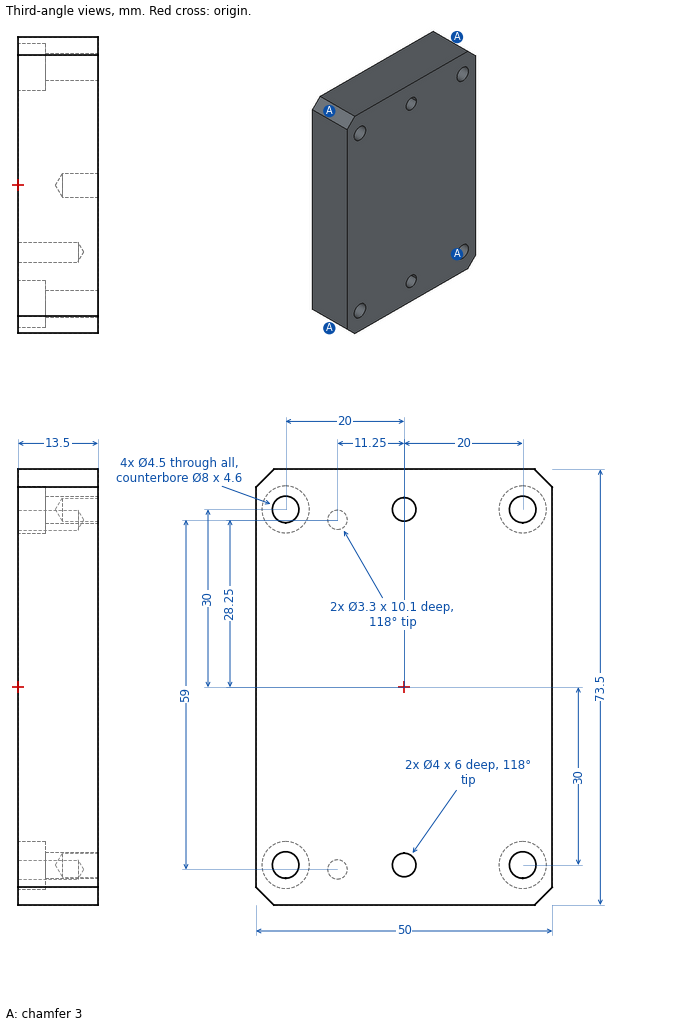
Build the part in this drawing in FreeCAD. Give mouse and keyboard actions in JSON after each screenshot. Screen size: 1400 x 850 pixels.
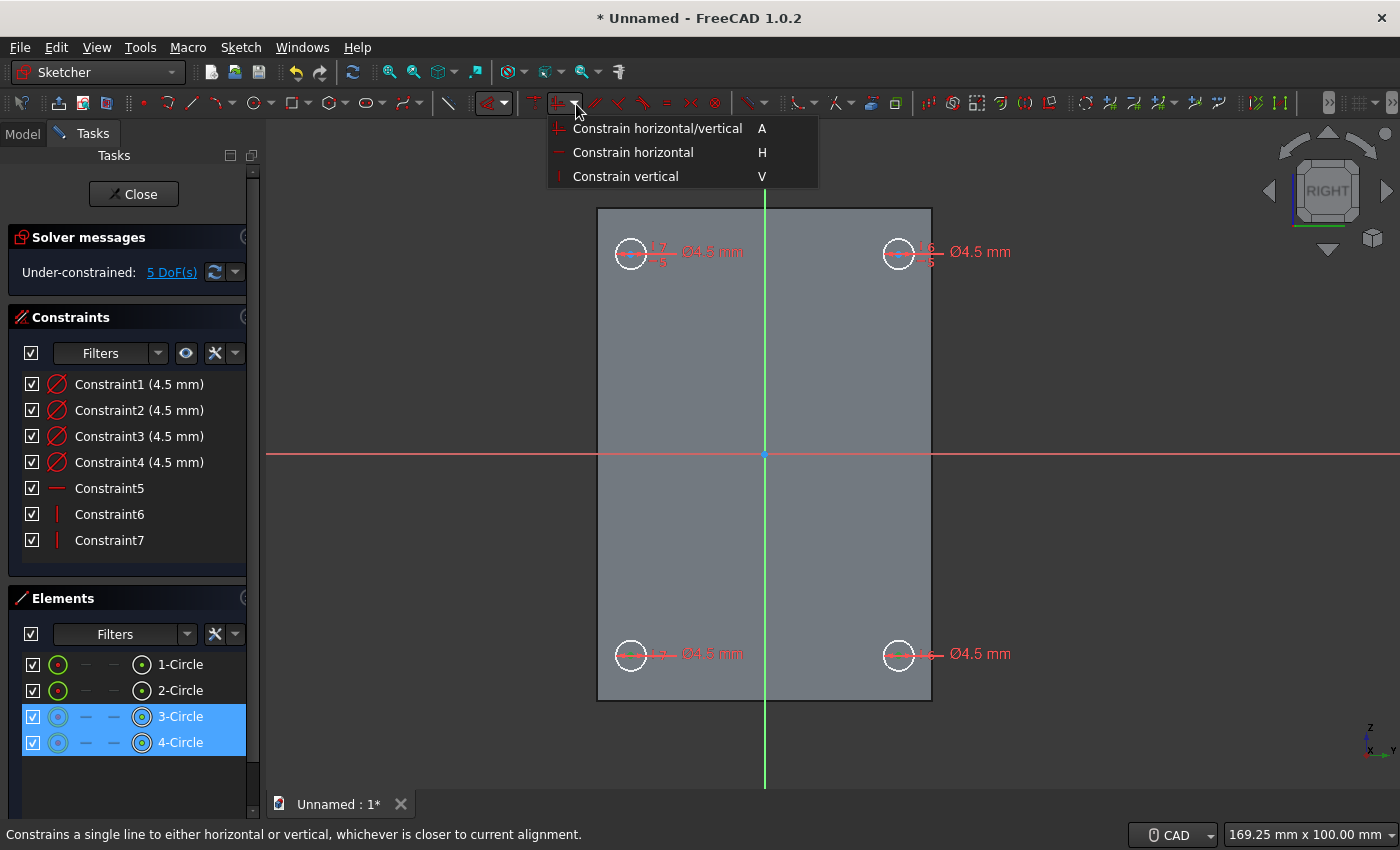
{"action": "left_click", "coordinate": [683, 152]}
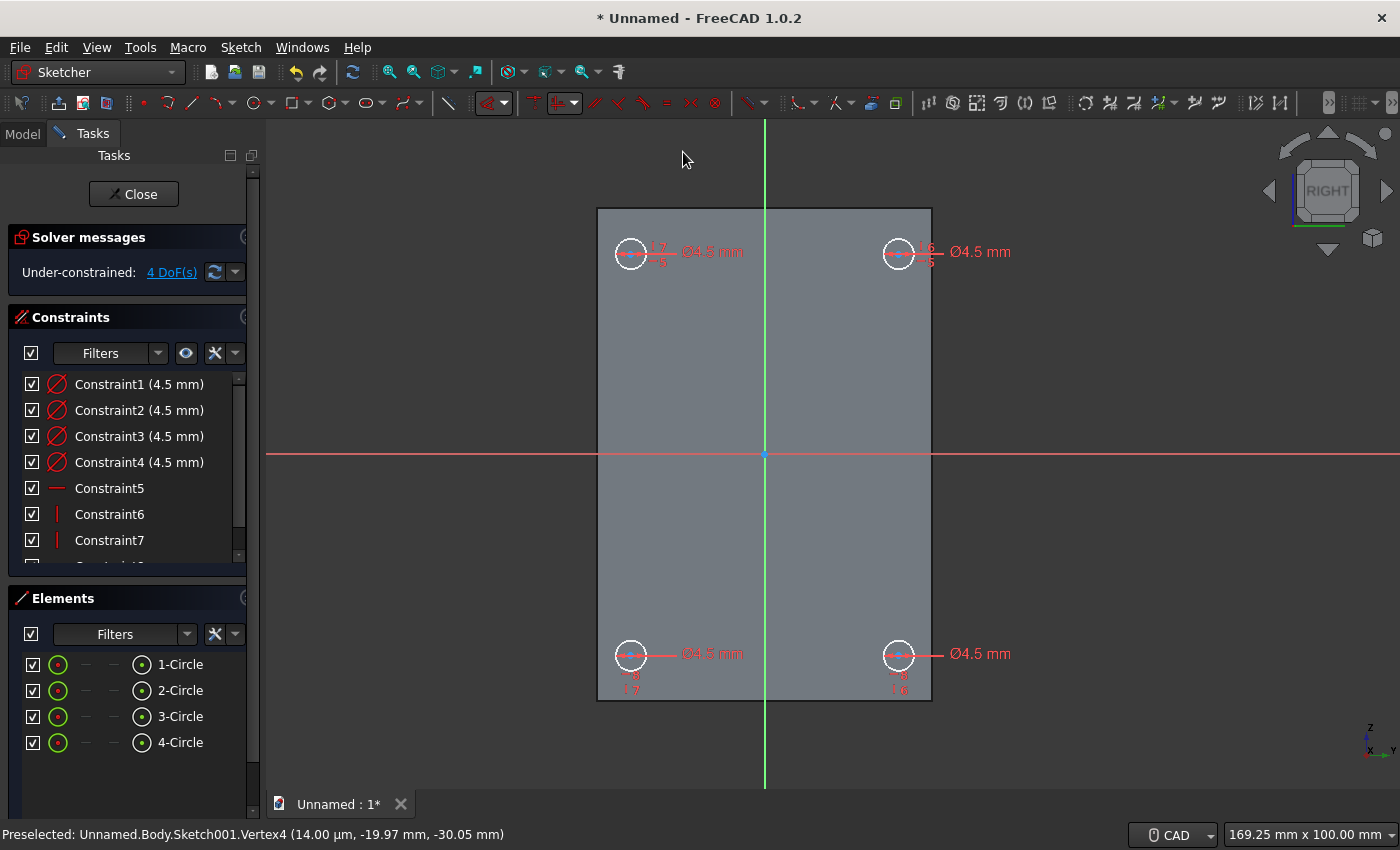
{"action": "left_click", "coordinate": [631, 254]}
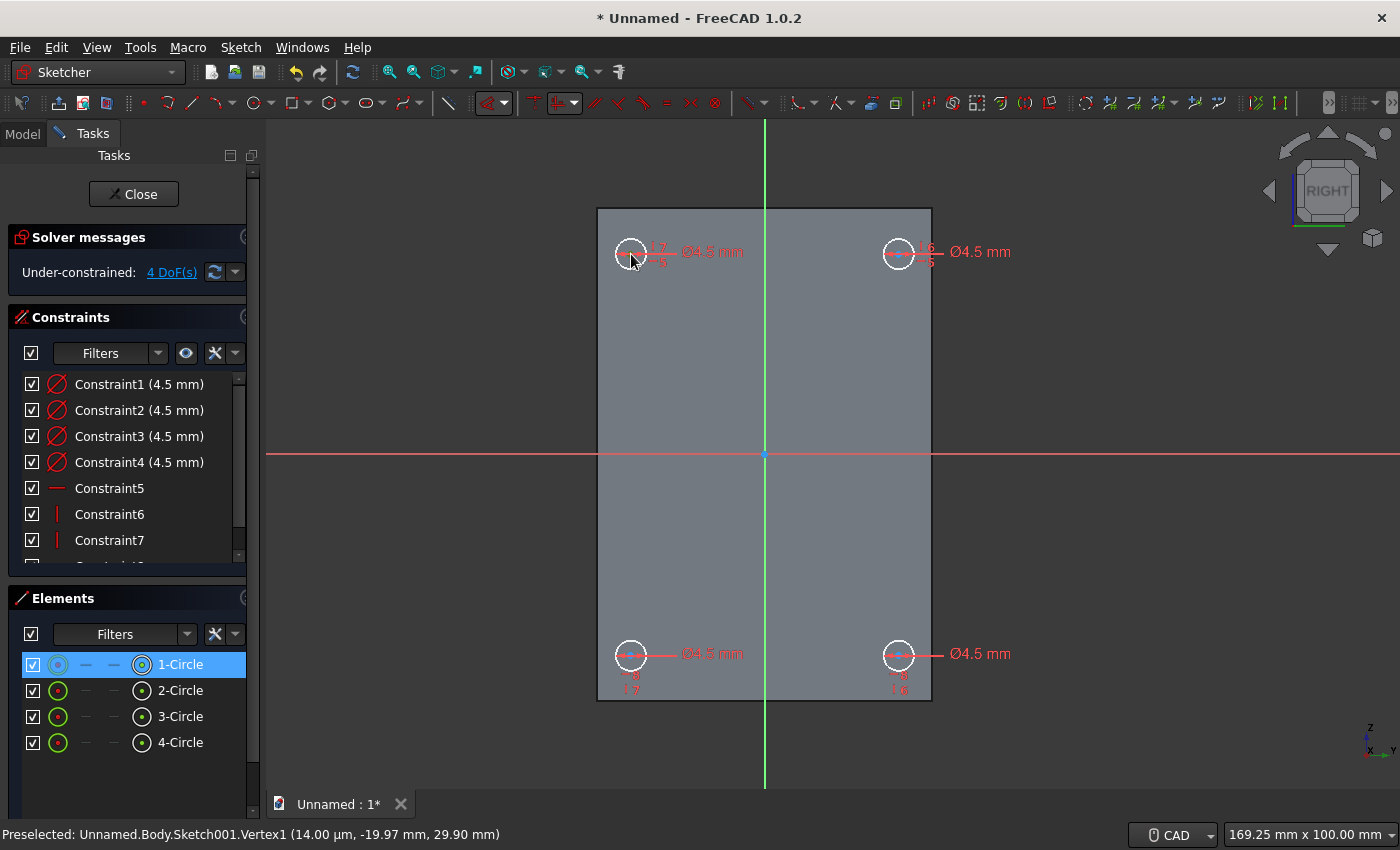
{"action": "left_click", "coordinate": [506, 104]}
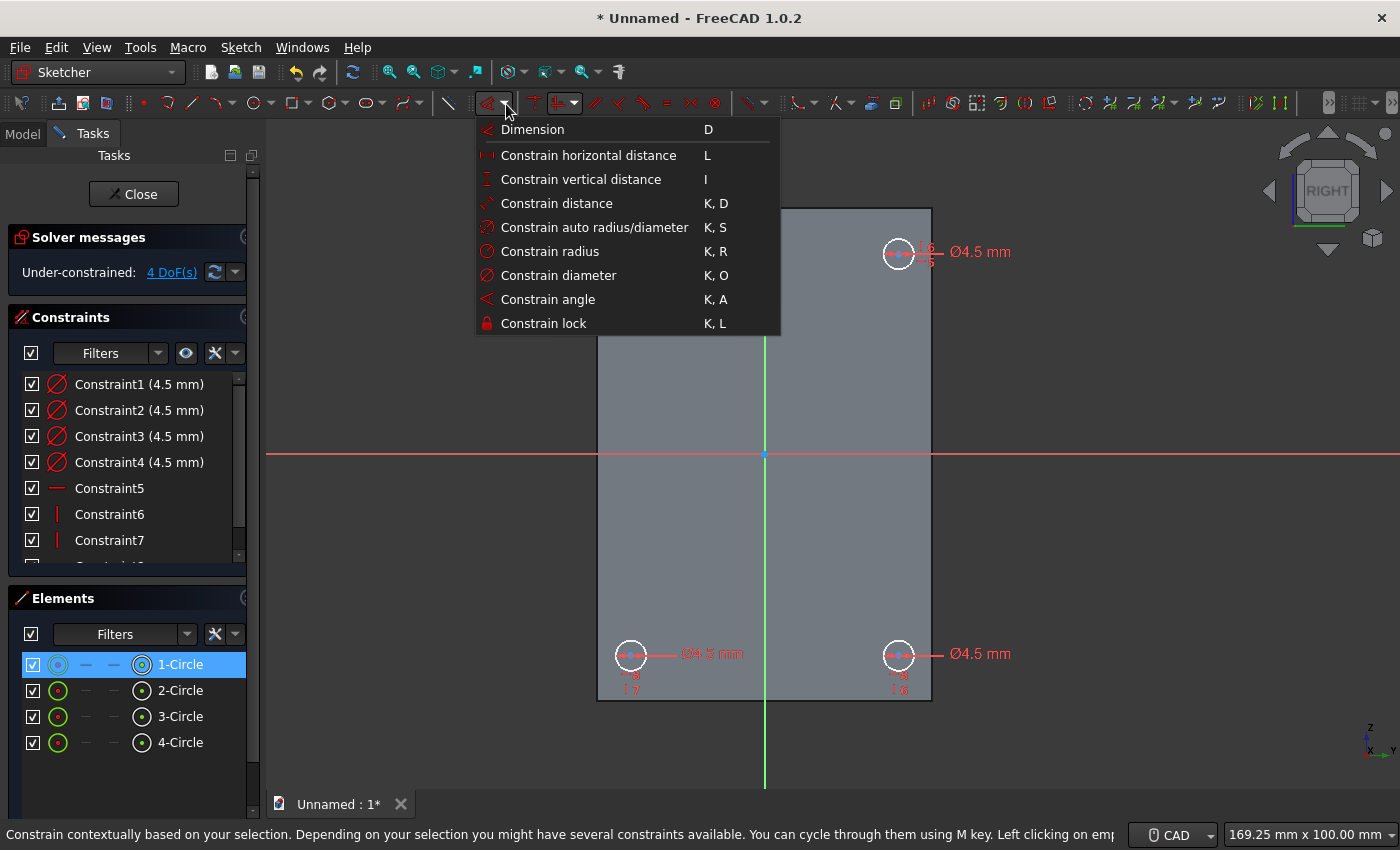
{"action": "left_click", "coordinate": [628, 155]}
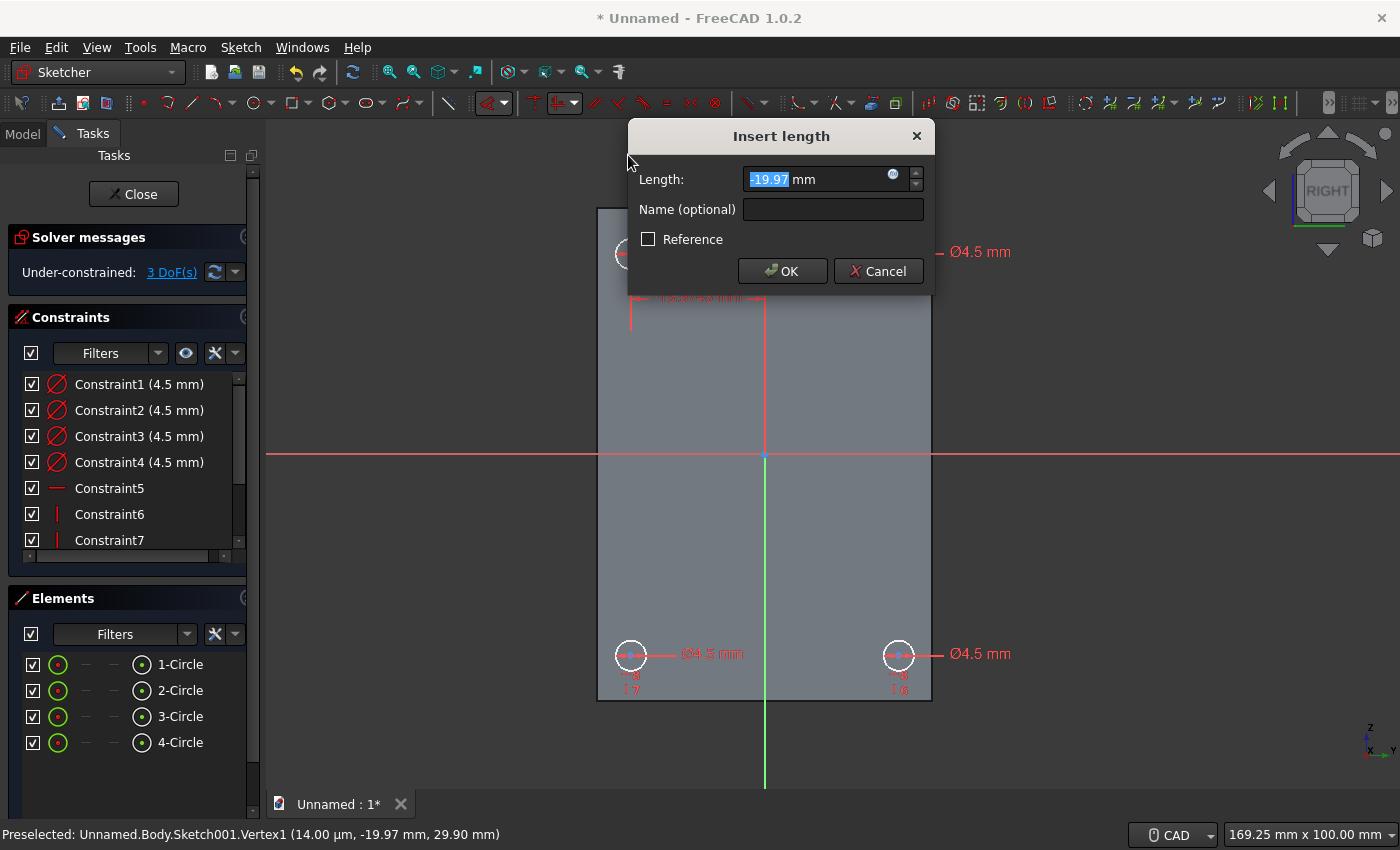
{"action": "type", "text": "-20"}
{"action": "key", "text": "Return"}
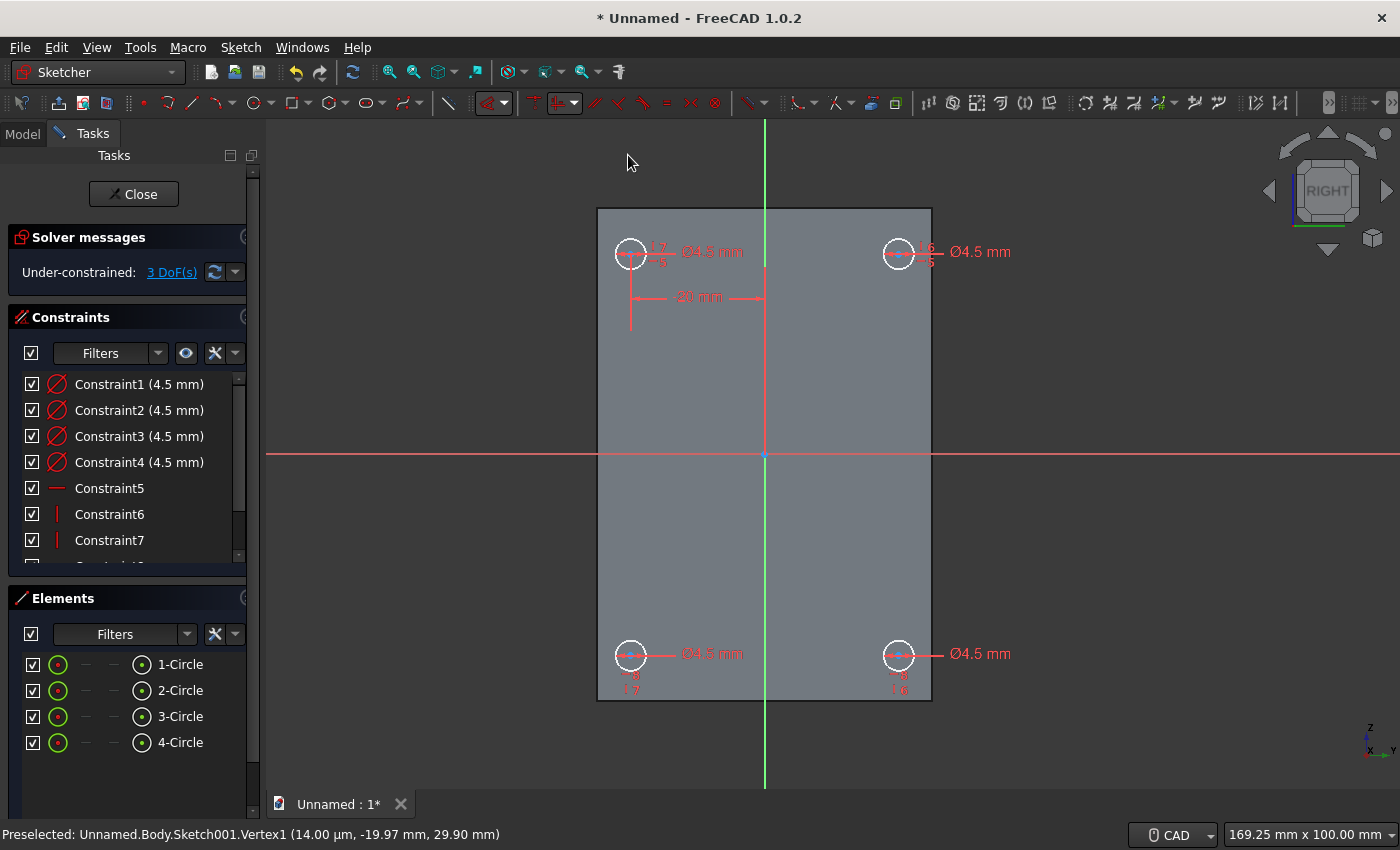
{"action": "left_click", "coordinate": [631, 254]}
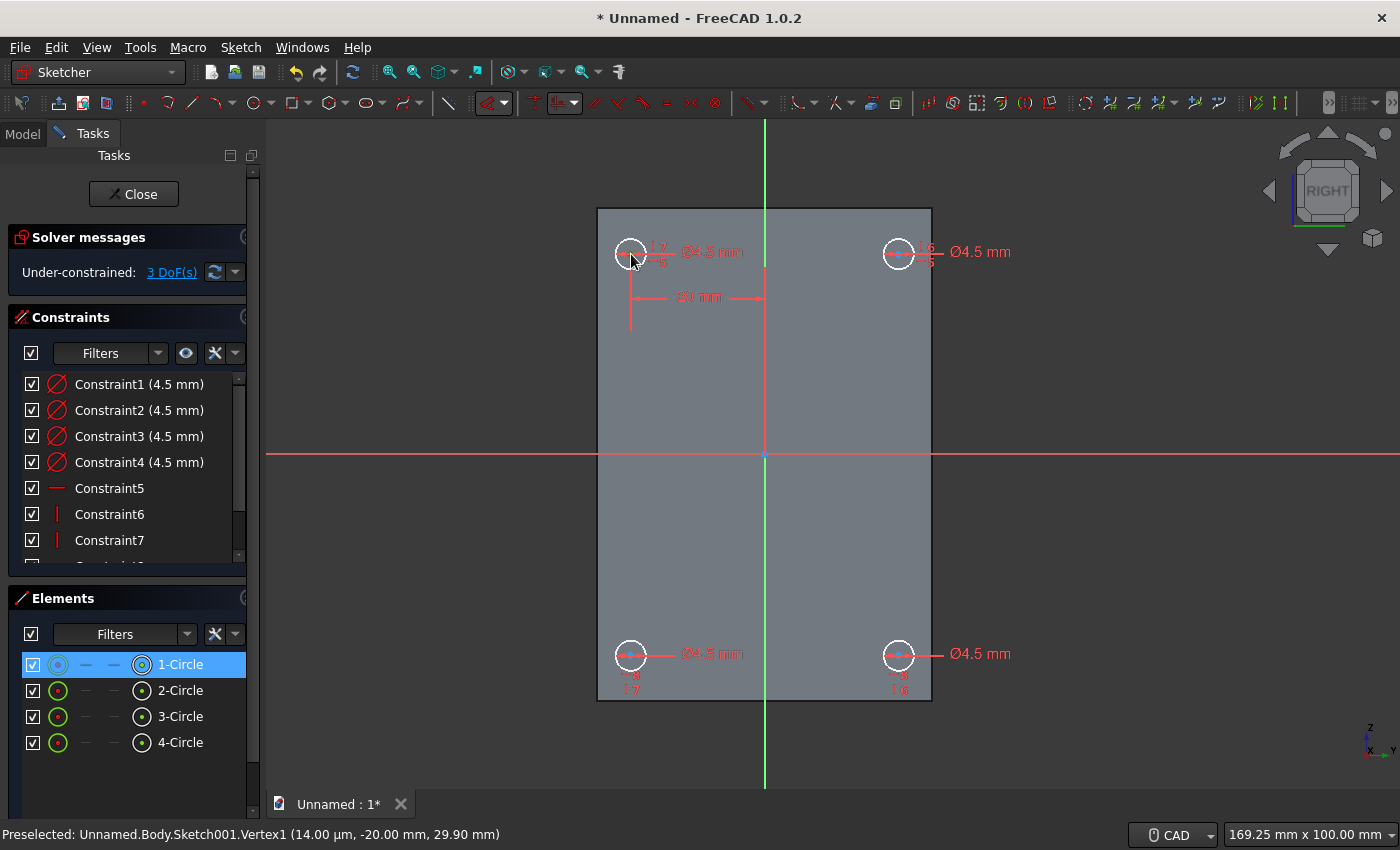
{"action": "left_click", "coordinate": [506, 104]}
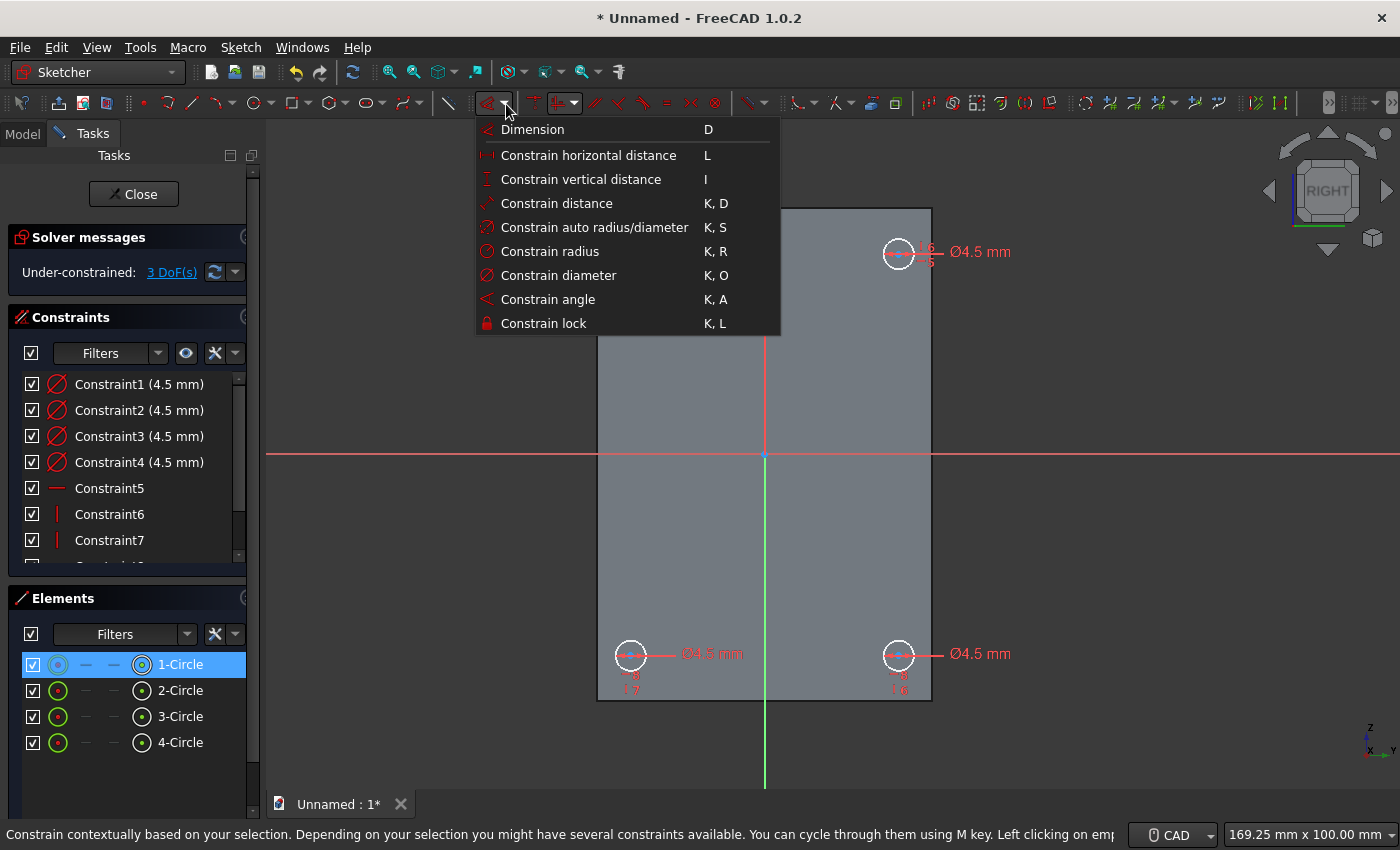
{"action": "left_click", "coordinate": [628, 179]}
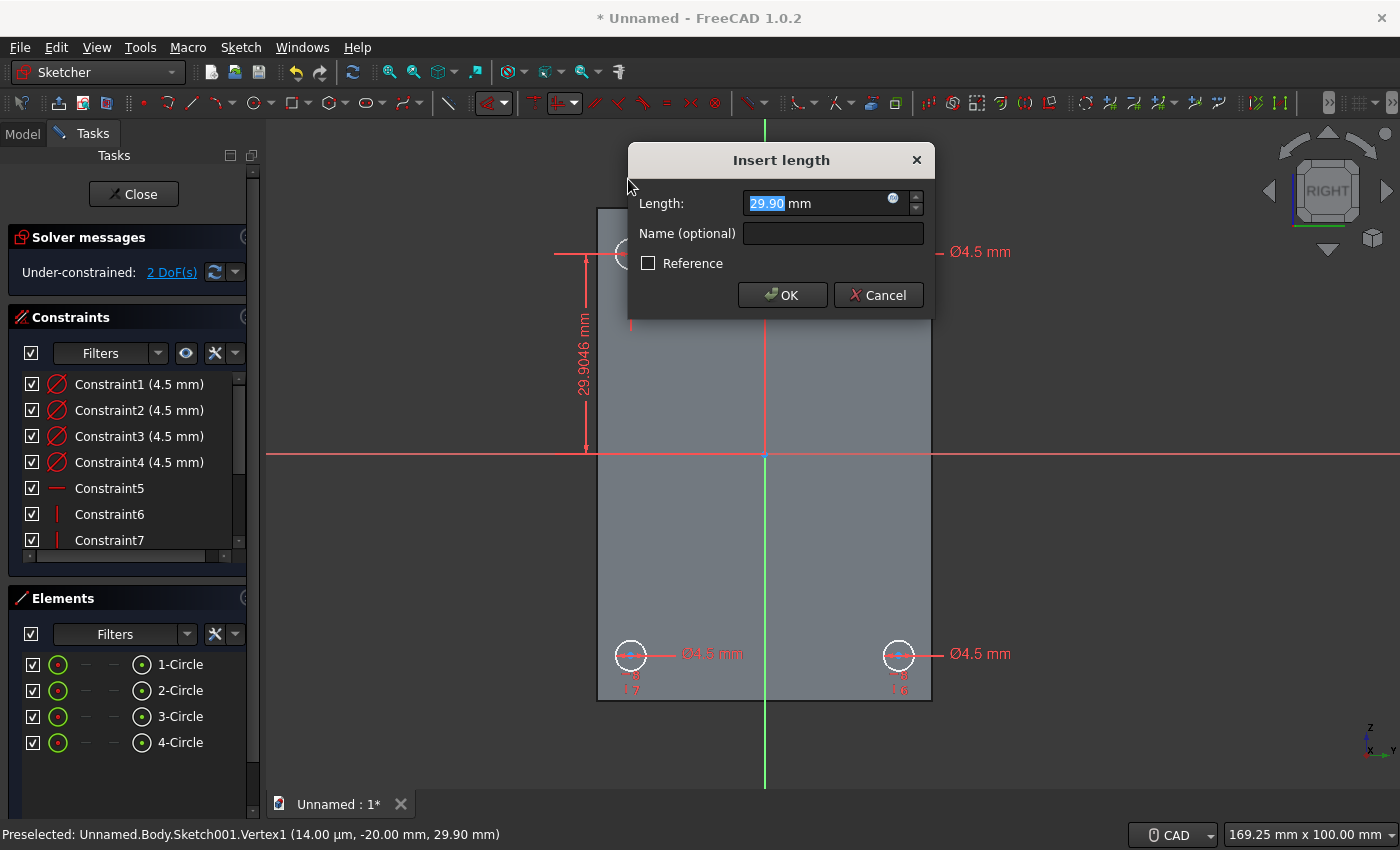
{"action": "type", "text": "30"}
{"action": "key", "text": "Return"}